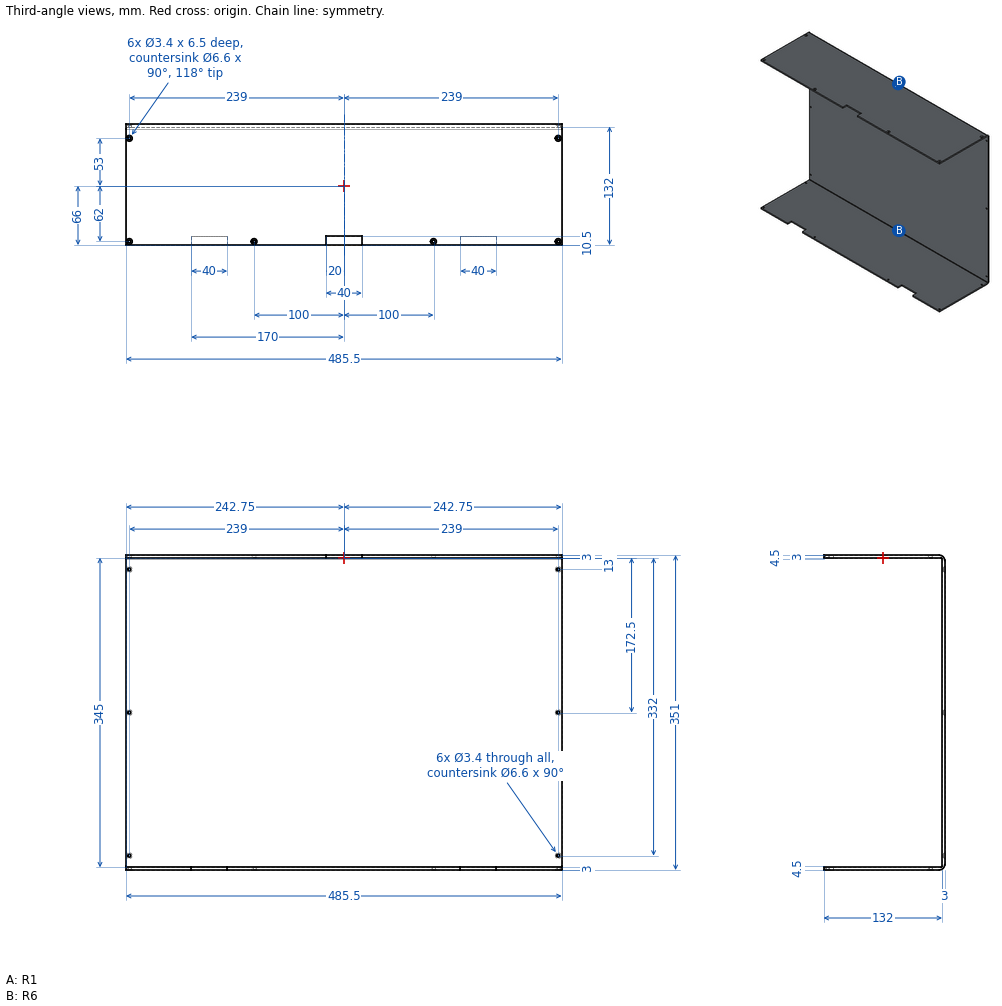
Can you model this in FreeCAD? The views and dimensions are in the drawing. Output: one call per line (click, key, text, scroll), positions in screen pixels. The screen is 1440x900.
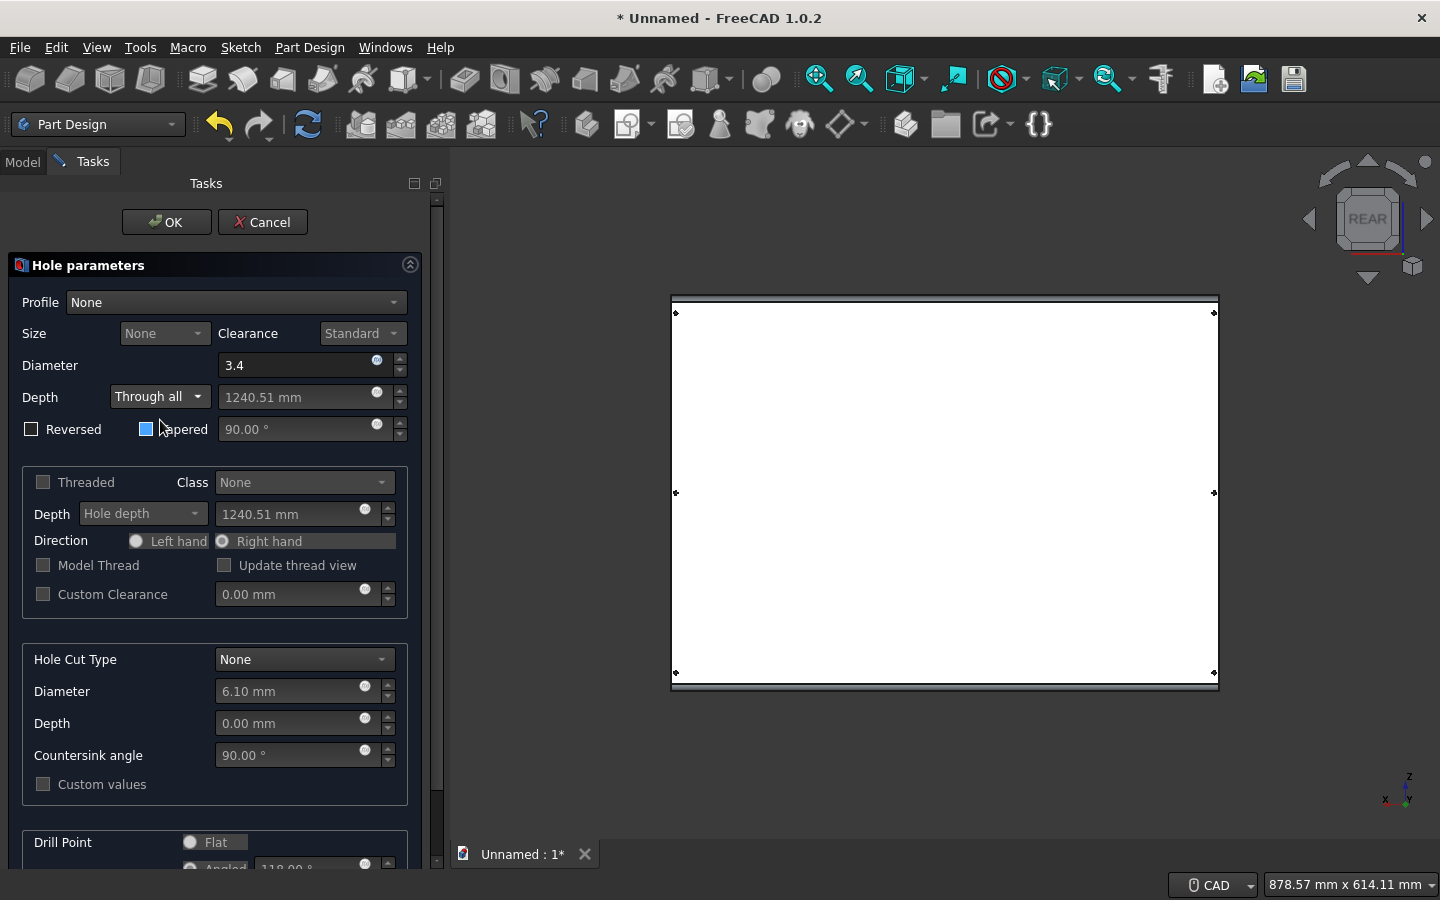
click(306, 660)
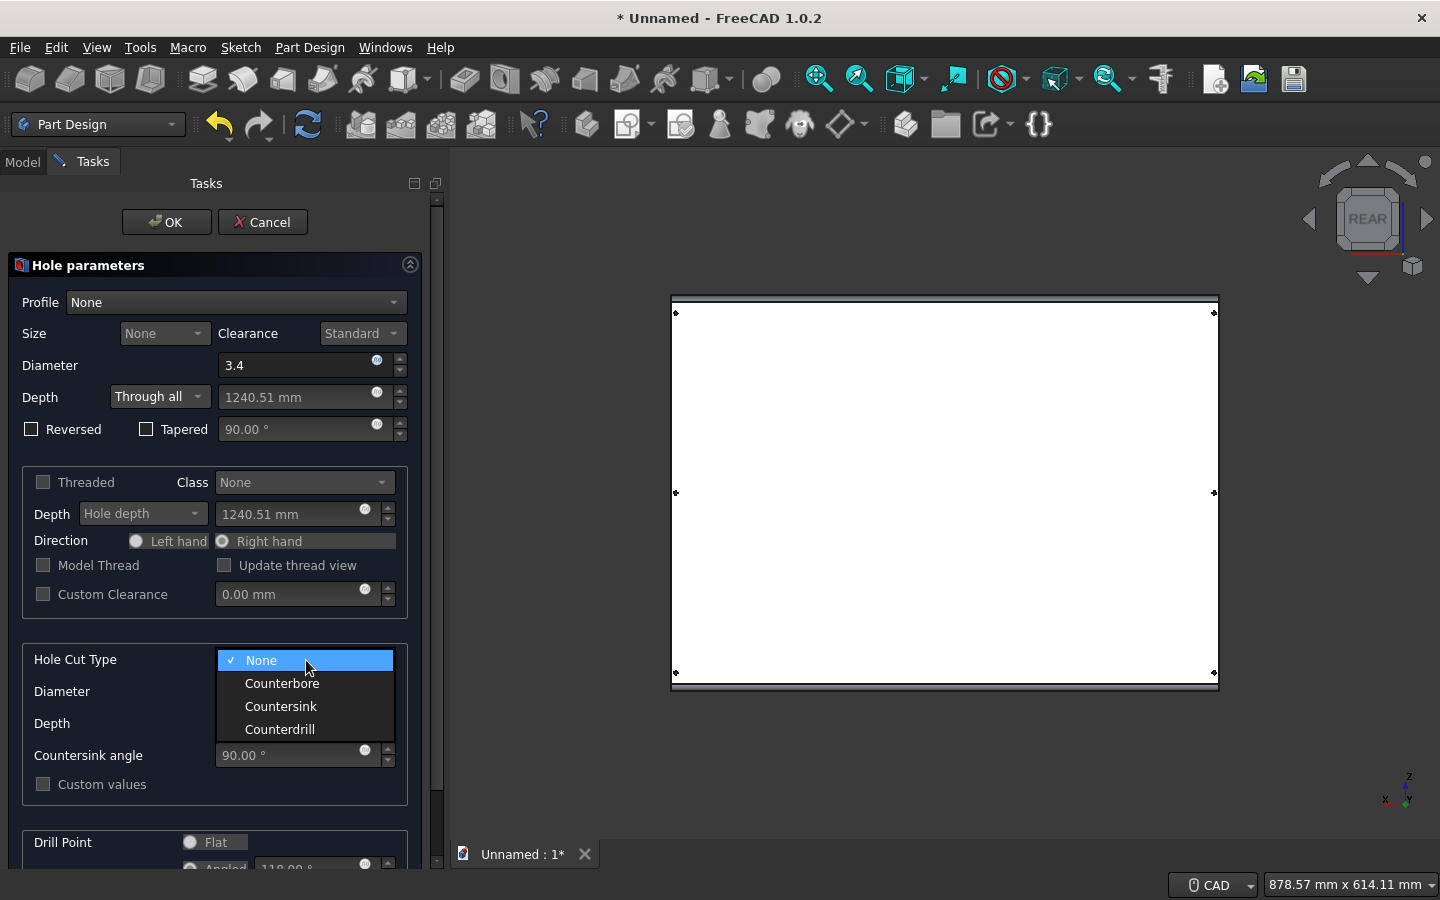
click(304, 706)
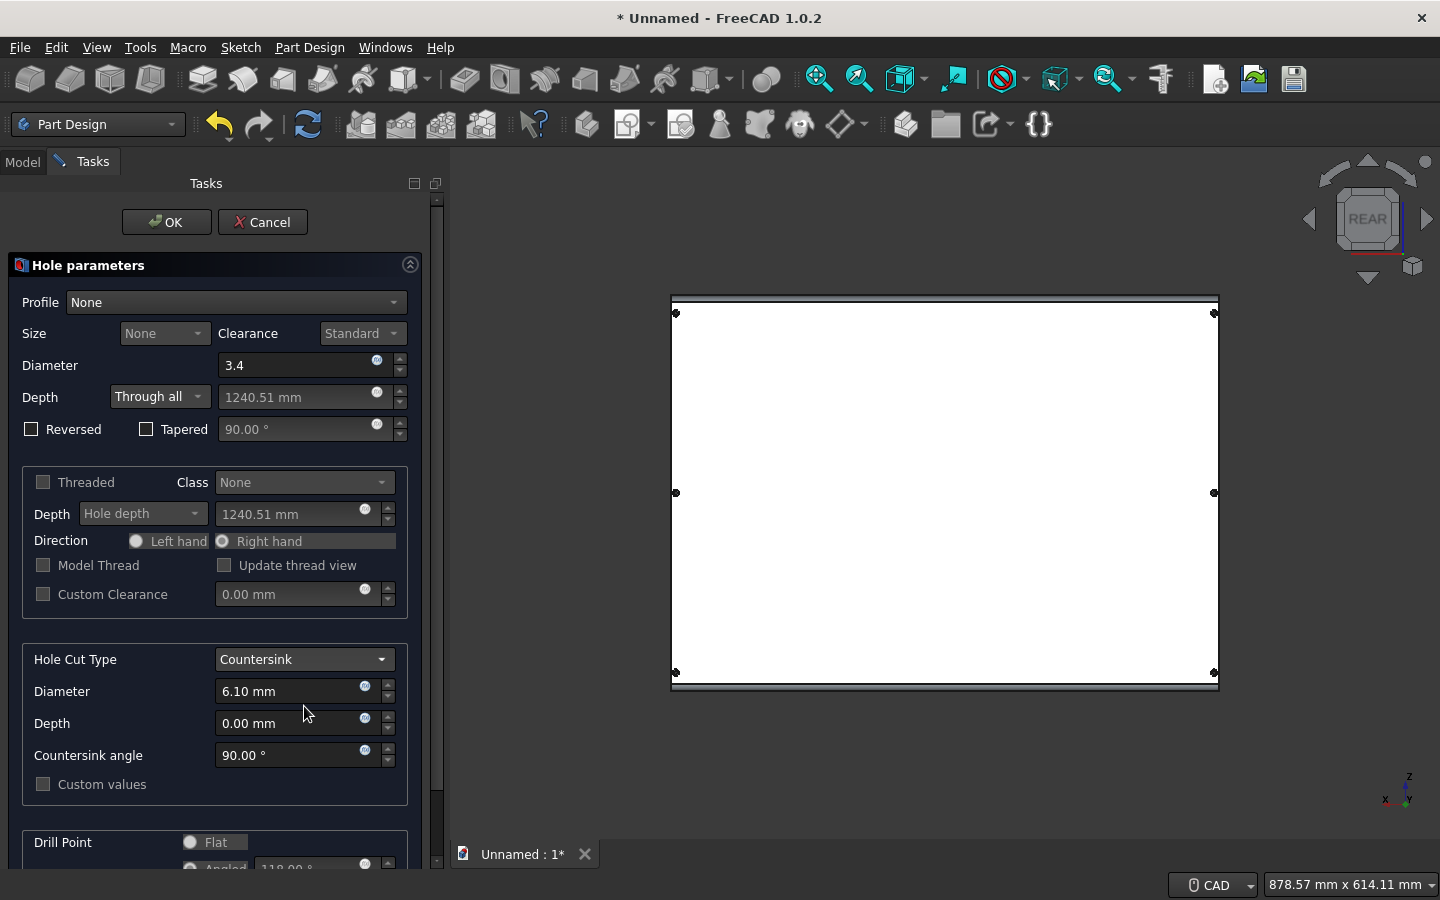
triple_click(298, 691)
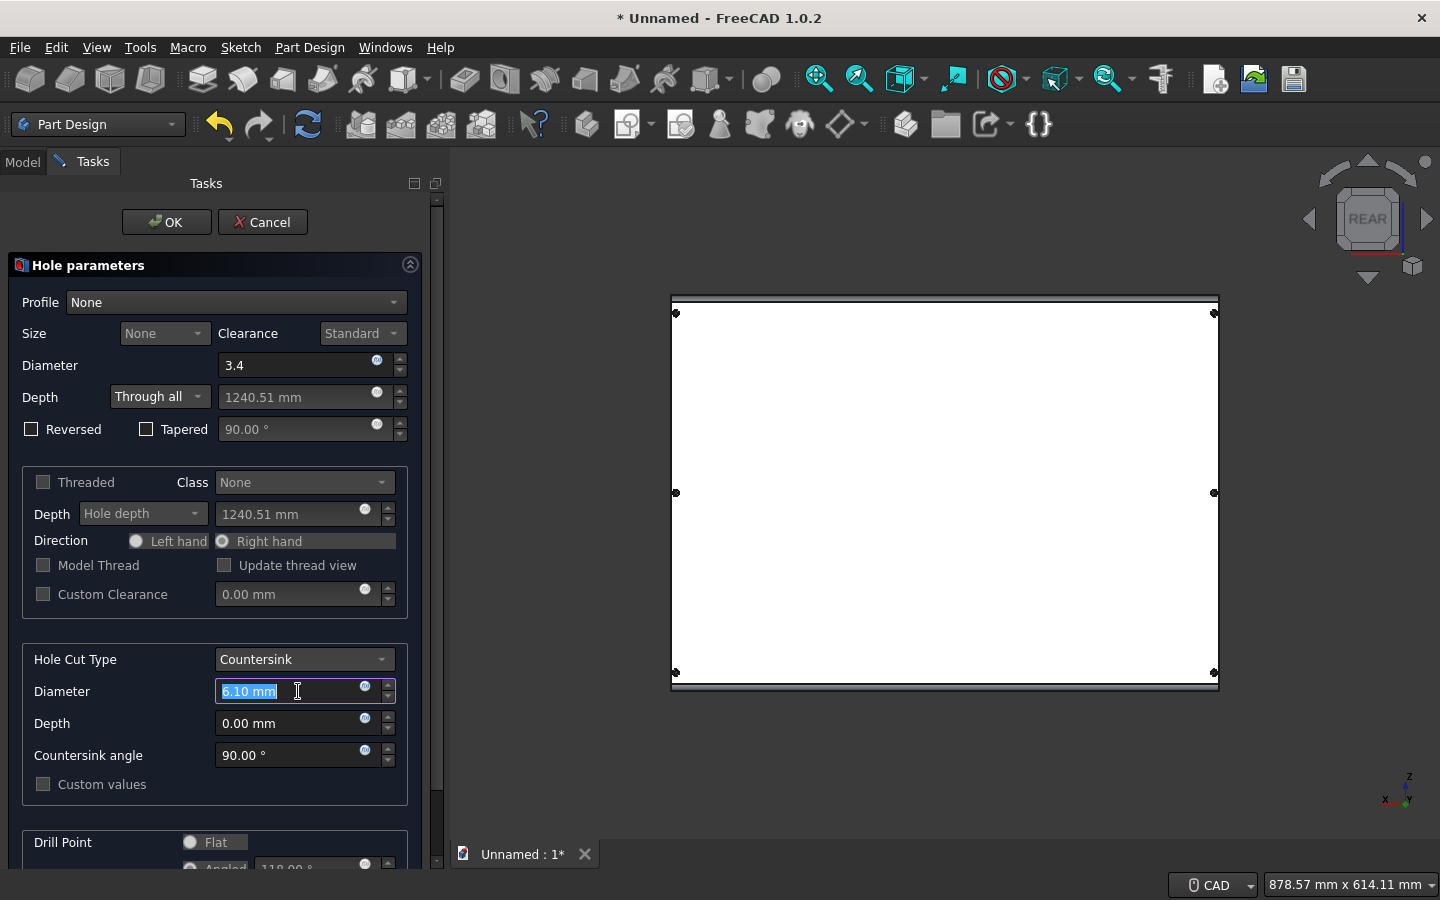
text(6.6)
key(Tab)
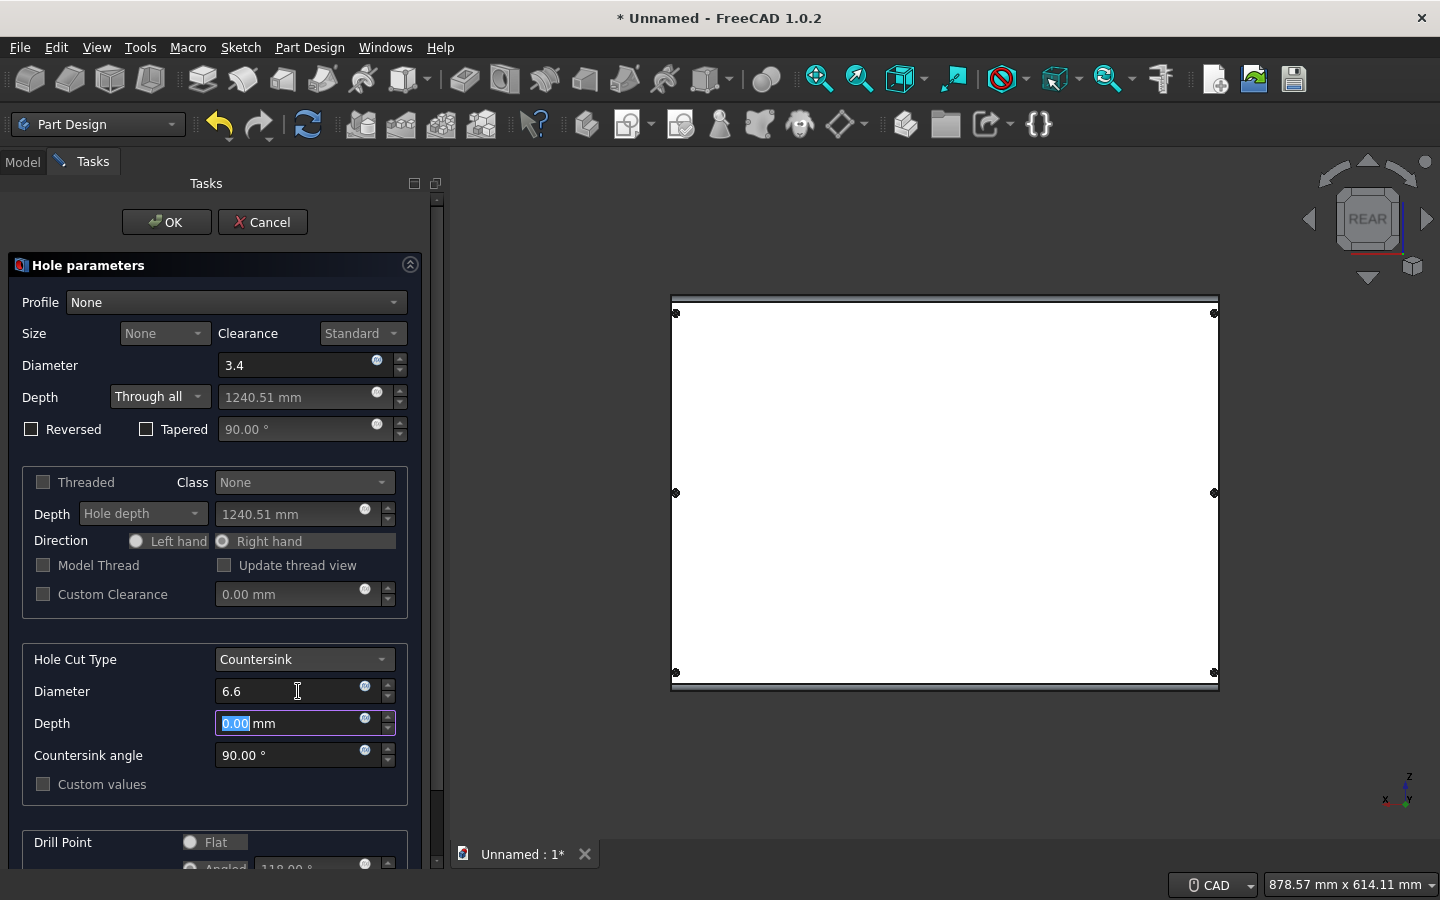
click(167, 222)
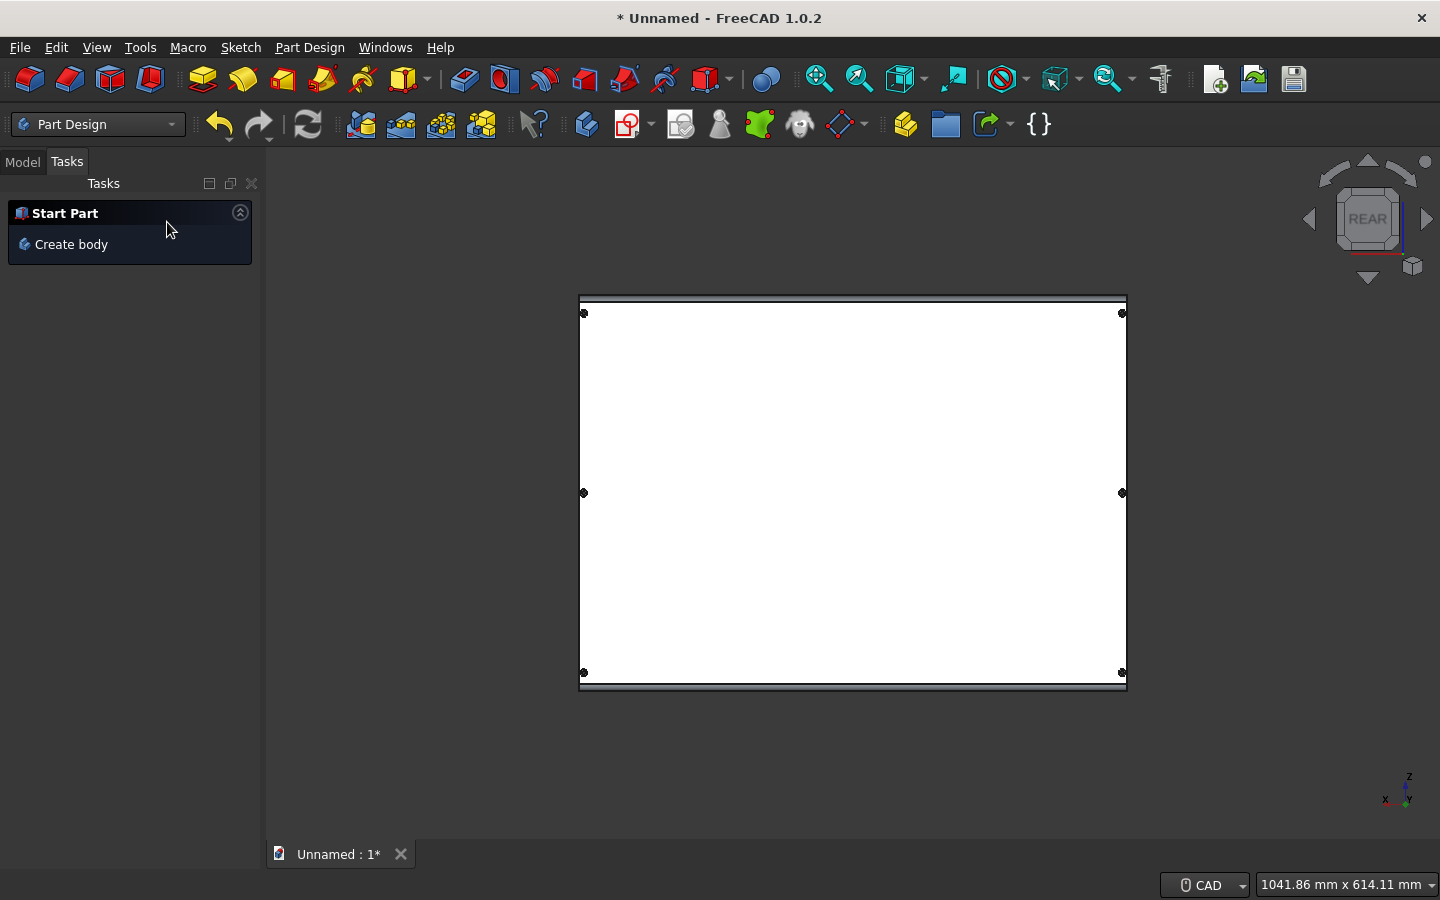
key(0)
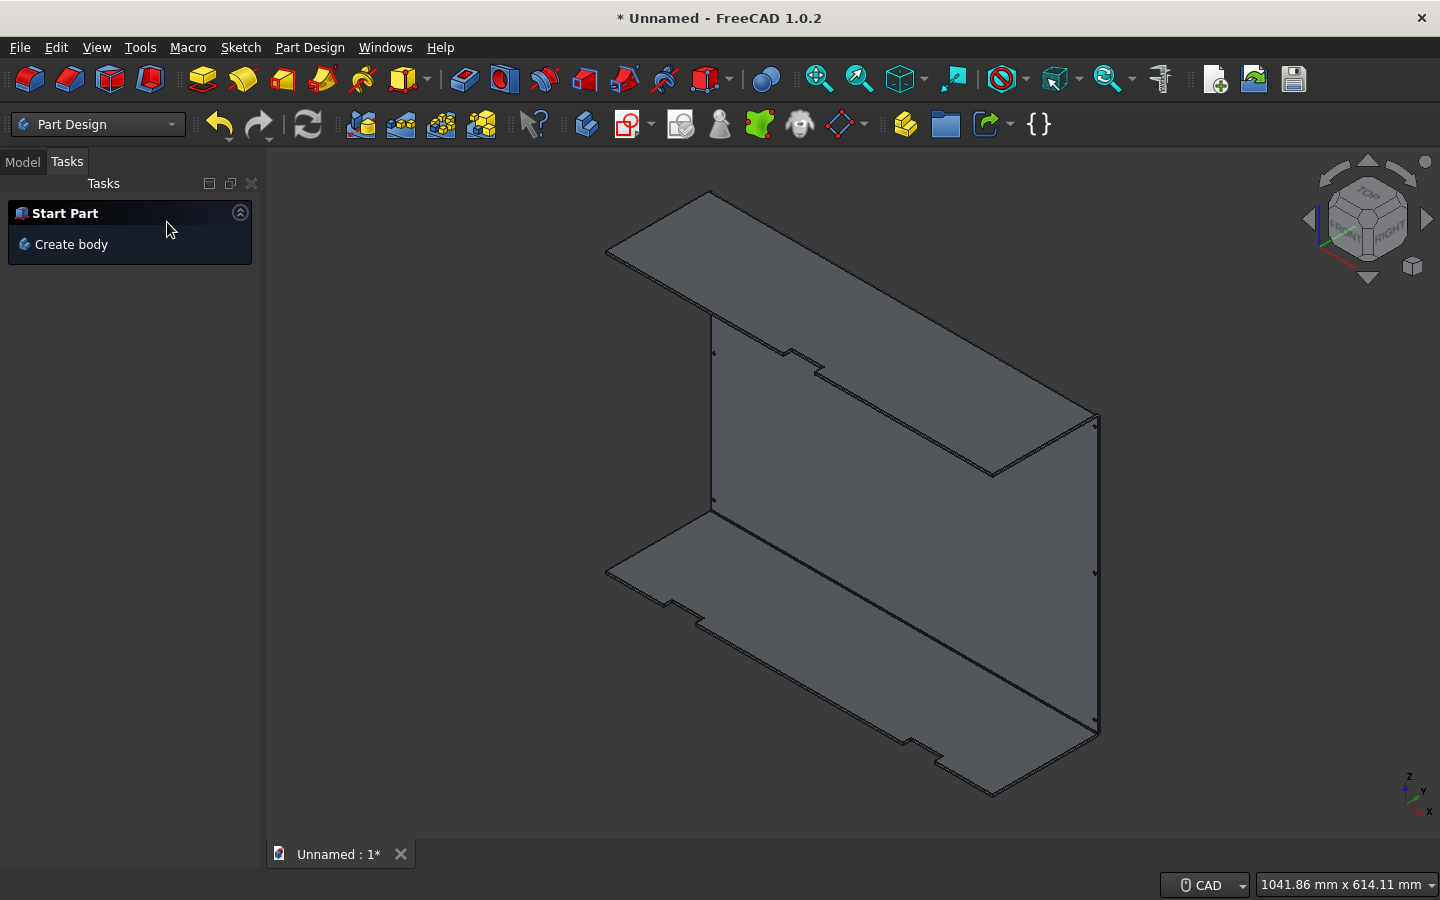
click(961, 396)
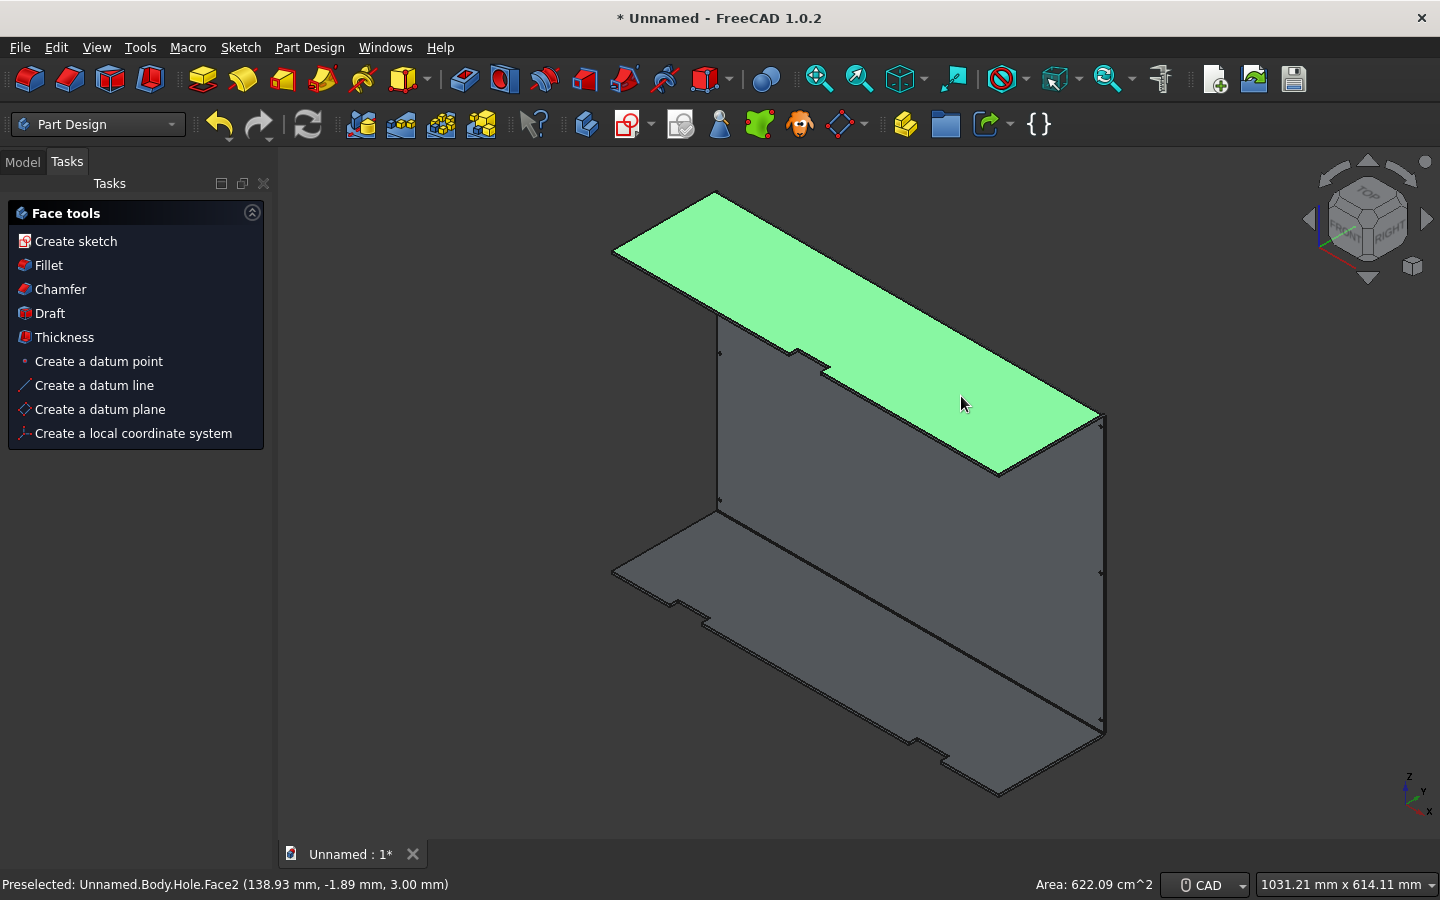
click(628, 124)